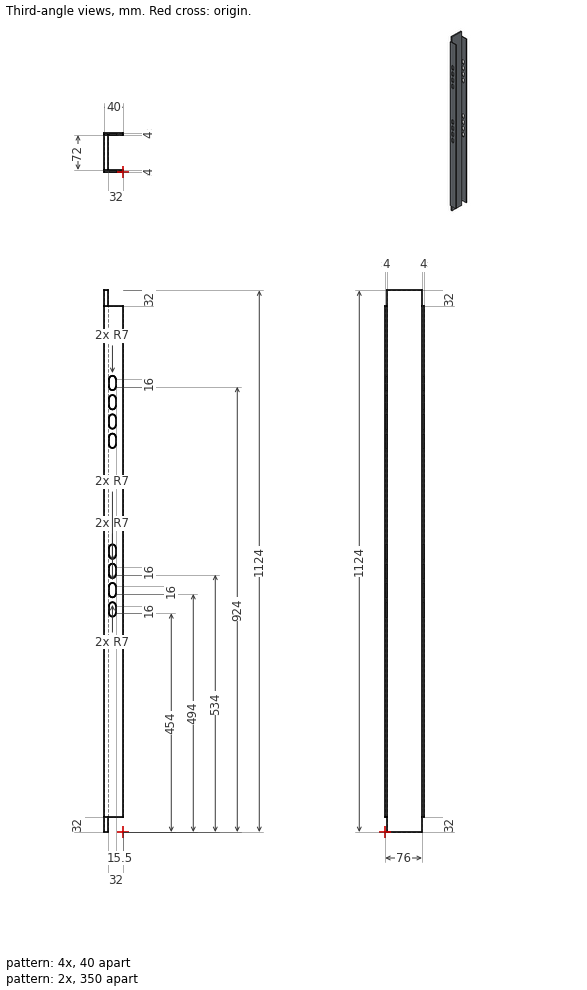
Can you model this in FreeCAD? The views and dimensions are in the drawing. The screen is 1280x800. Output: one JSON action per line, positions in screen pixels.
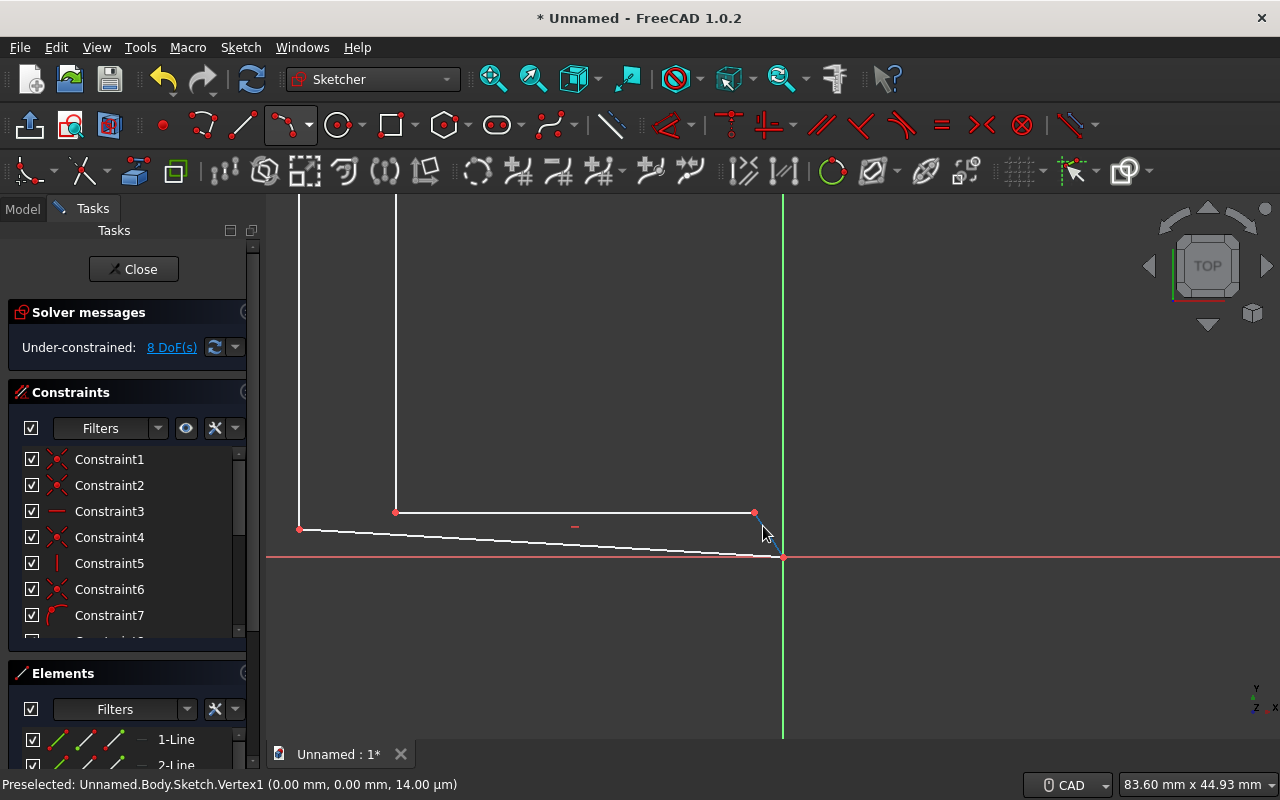
{"action": "left_click", "coordinate": [763, 526]}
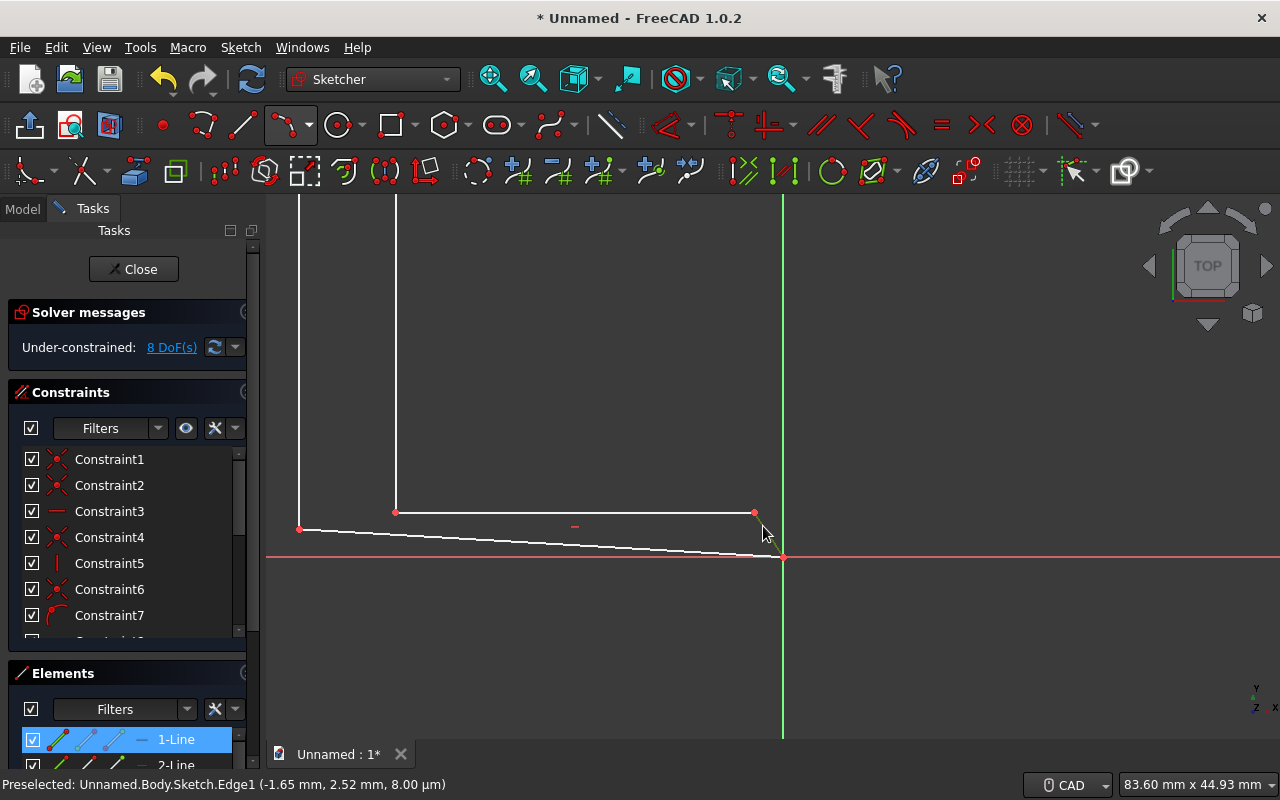
{"action": "left_click", "coordinate": [796, 126]}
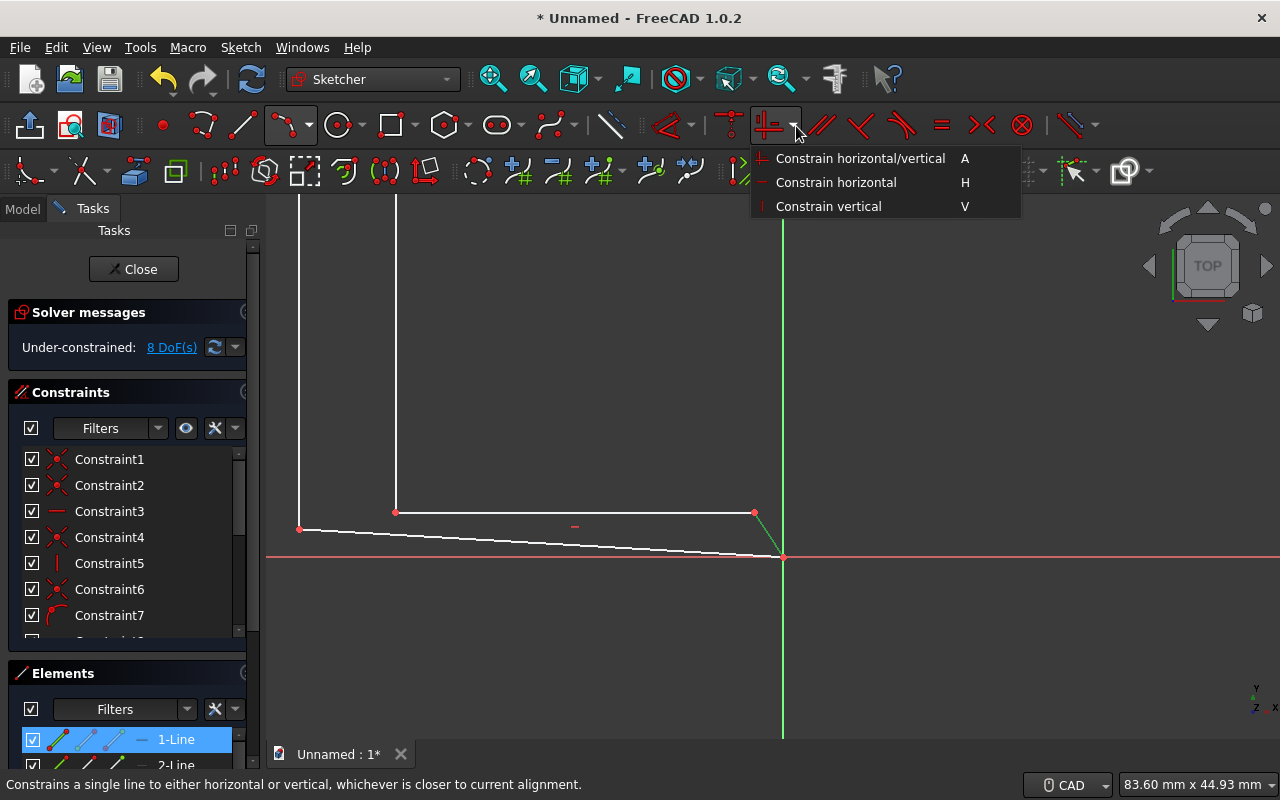
{"action": "left_click", "coordinate": [886, 206]}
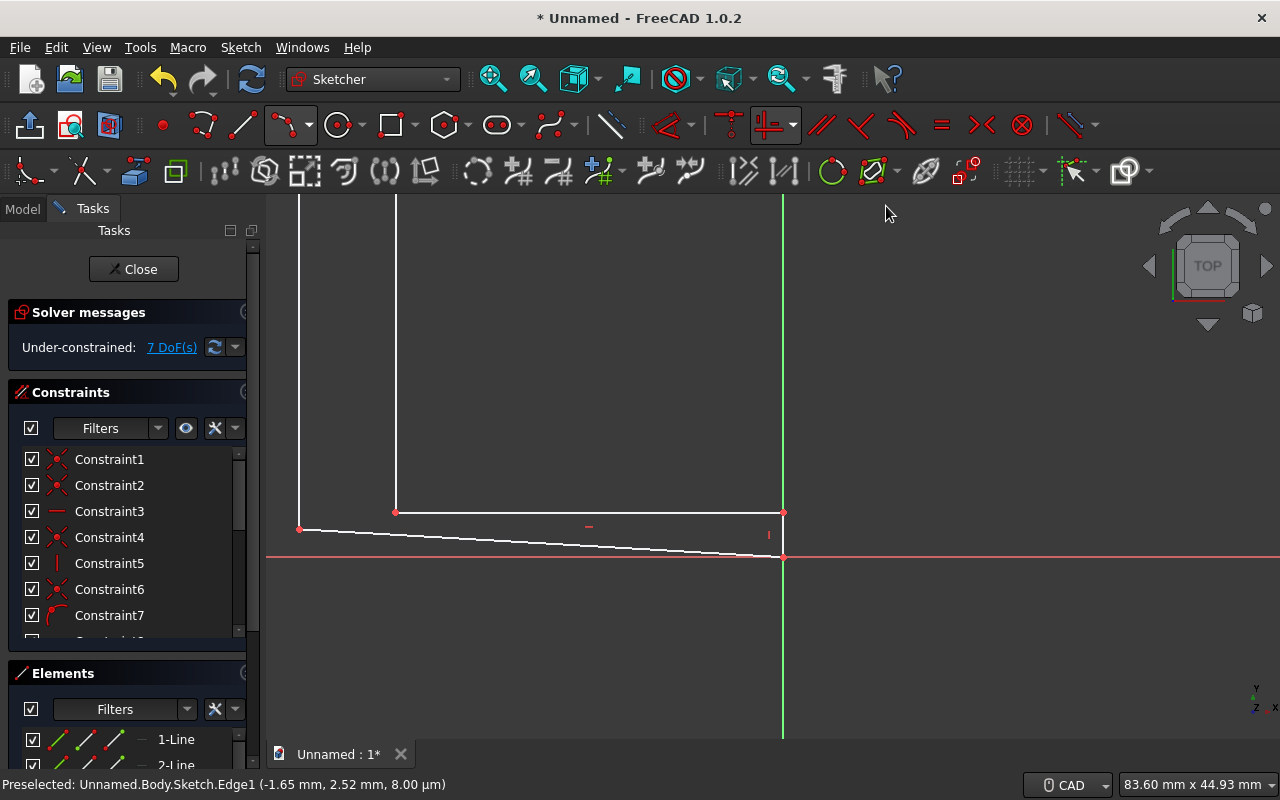
{"action": "scroll", "coordinate": [800, 696], "scroll_direction": "down", "scroll_amount": 5}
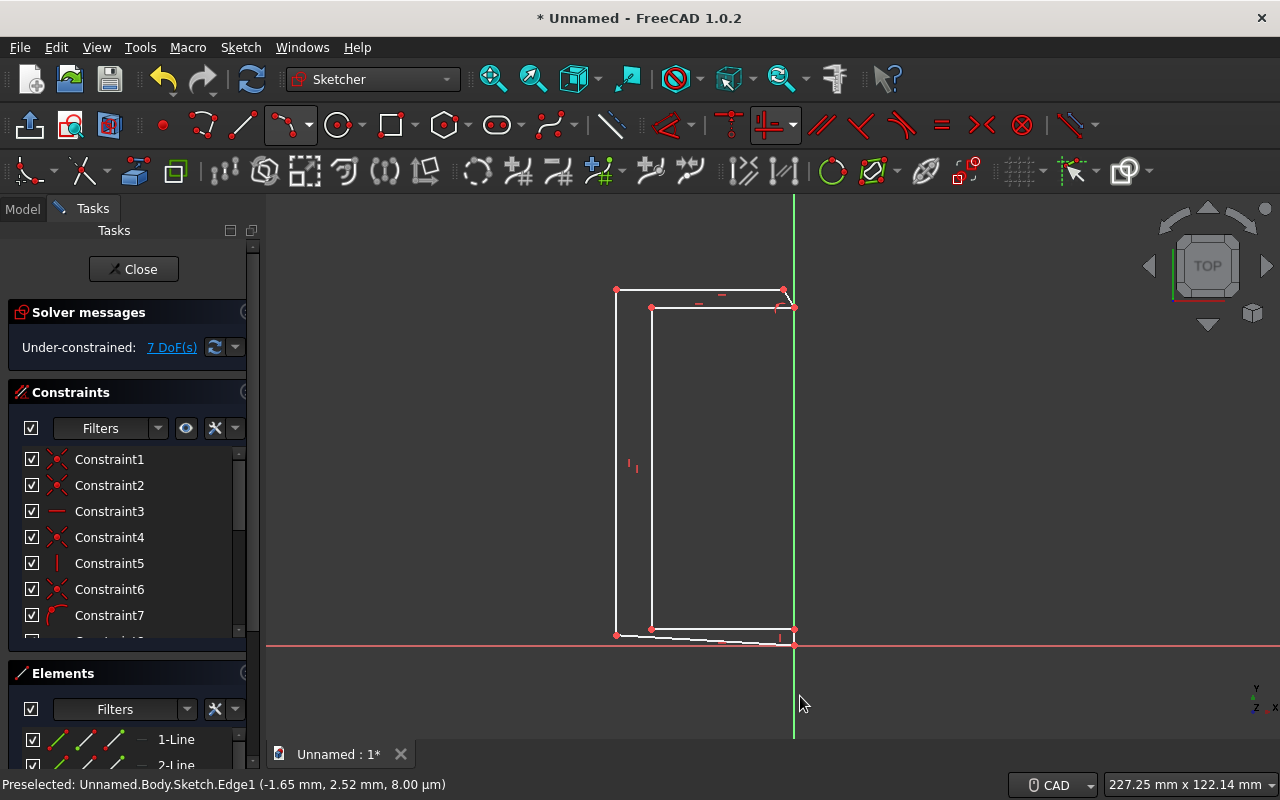
{"action": "scroll", "coordinate": [787, 295], "scroll_direction": "up", "scroll_amount": 4}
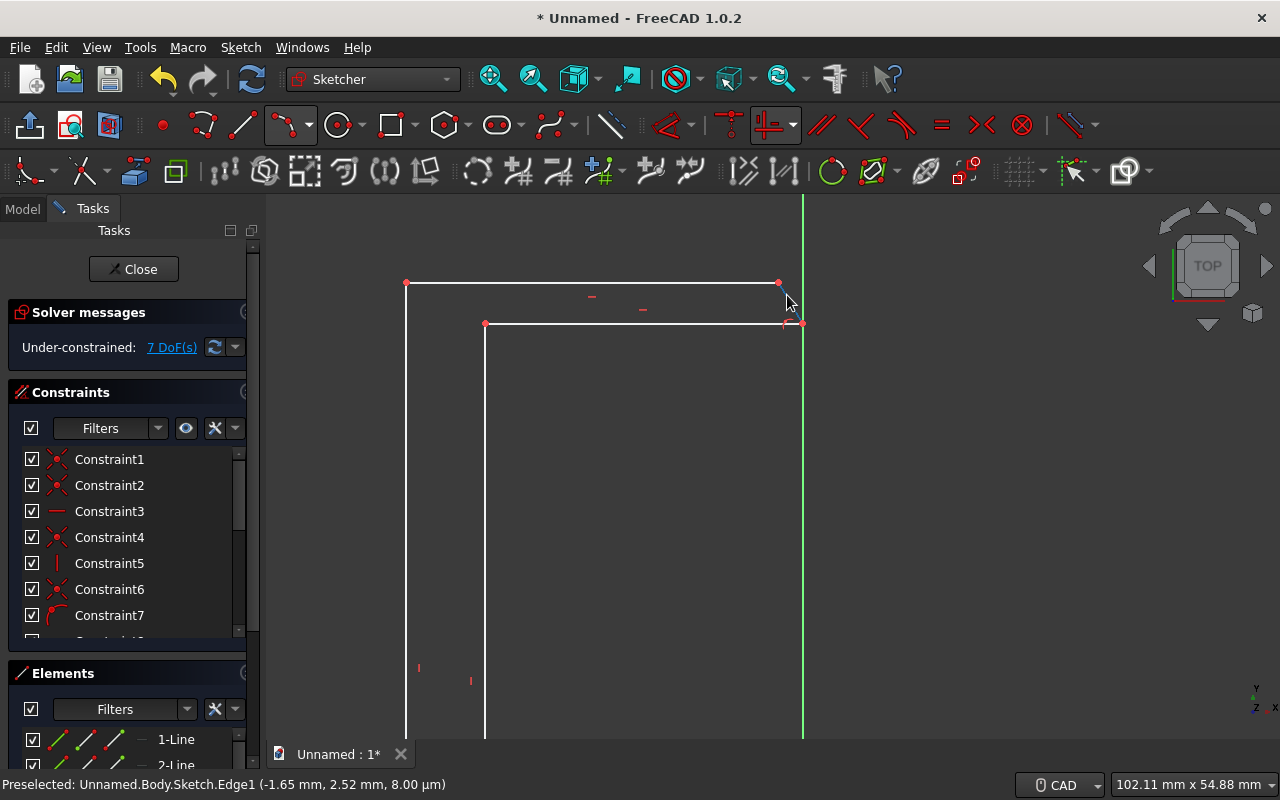
{"action": "left_click", "coordinate": [786, 295]}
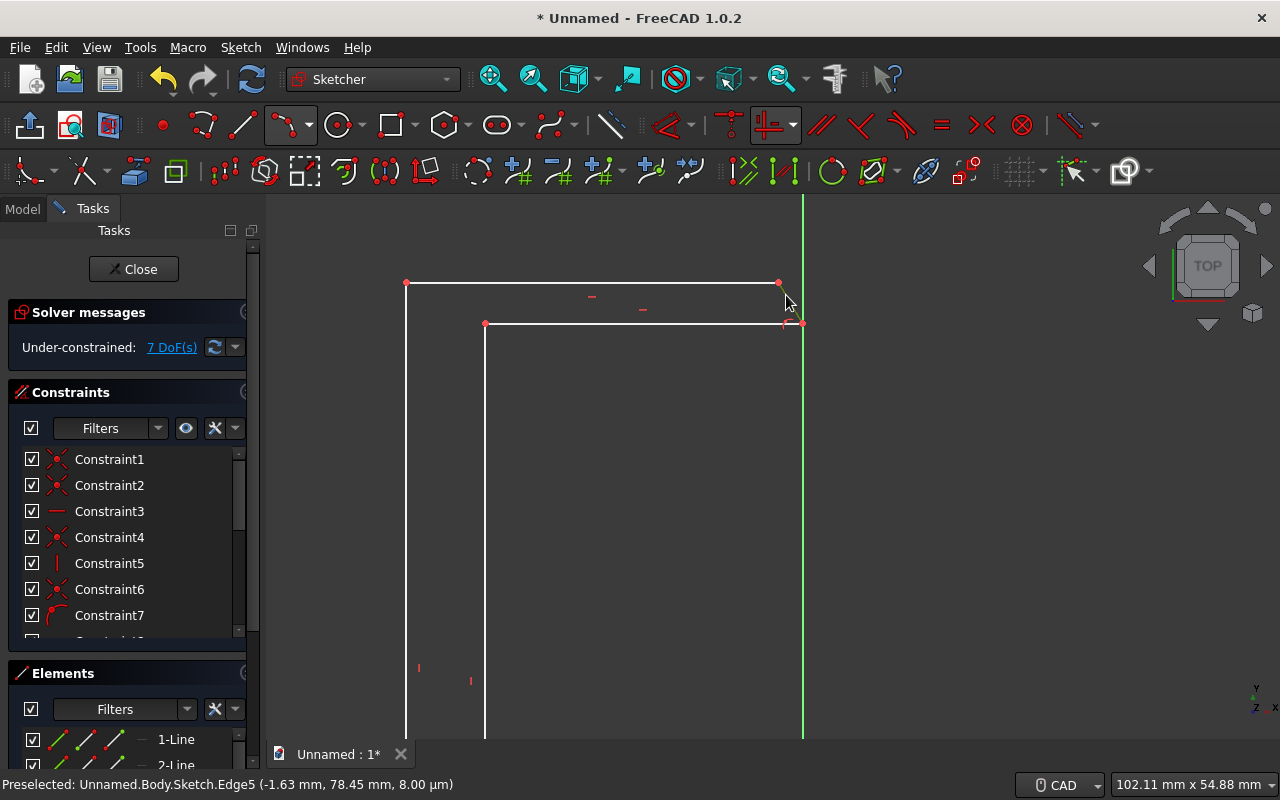
{"action": "left_click", "coordinate": [796, 126]}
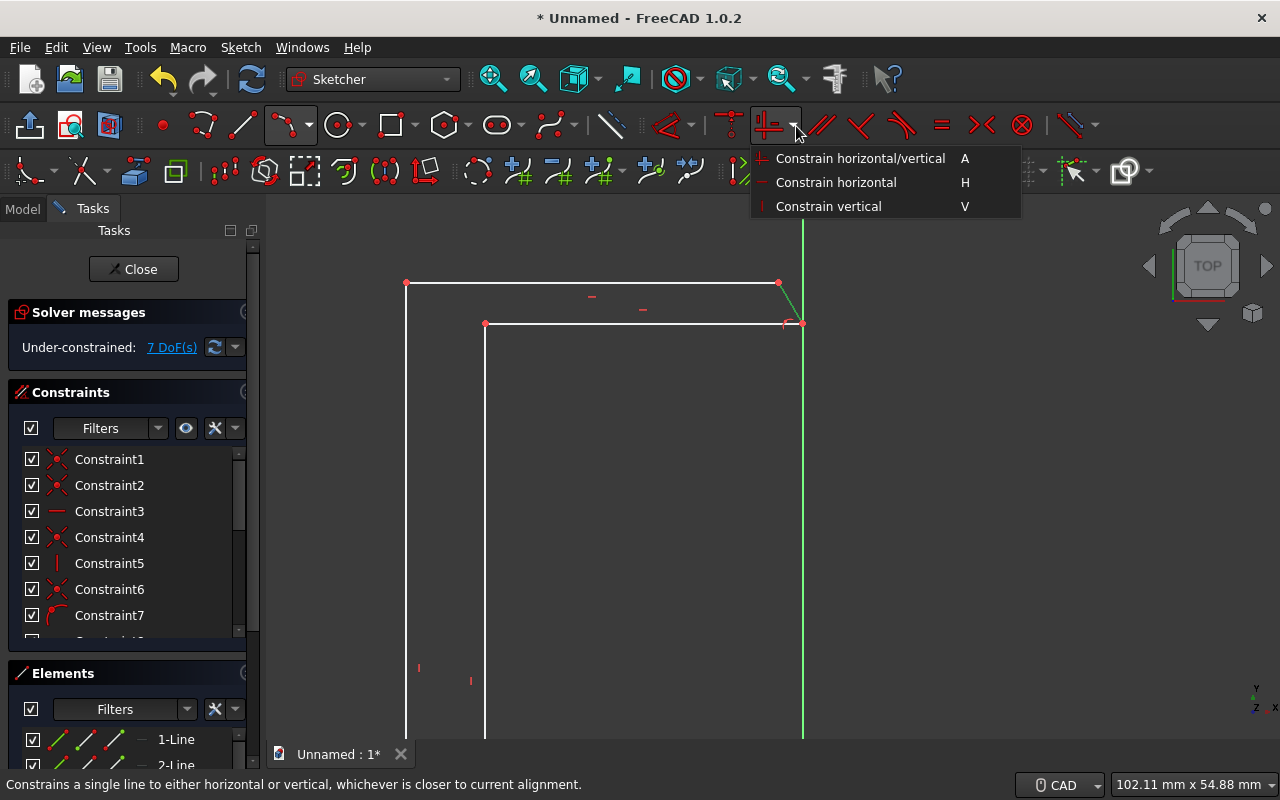
{"action": "left_click", "coordinate": [886, 206]}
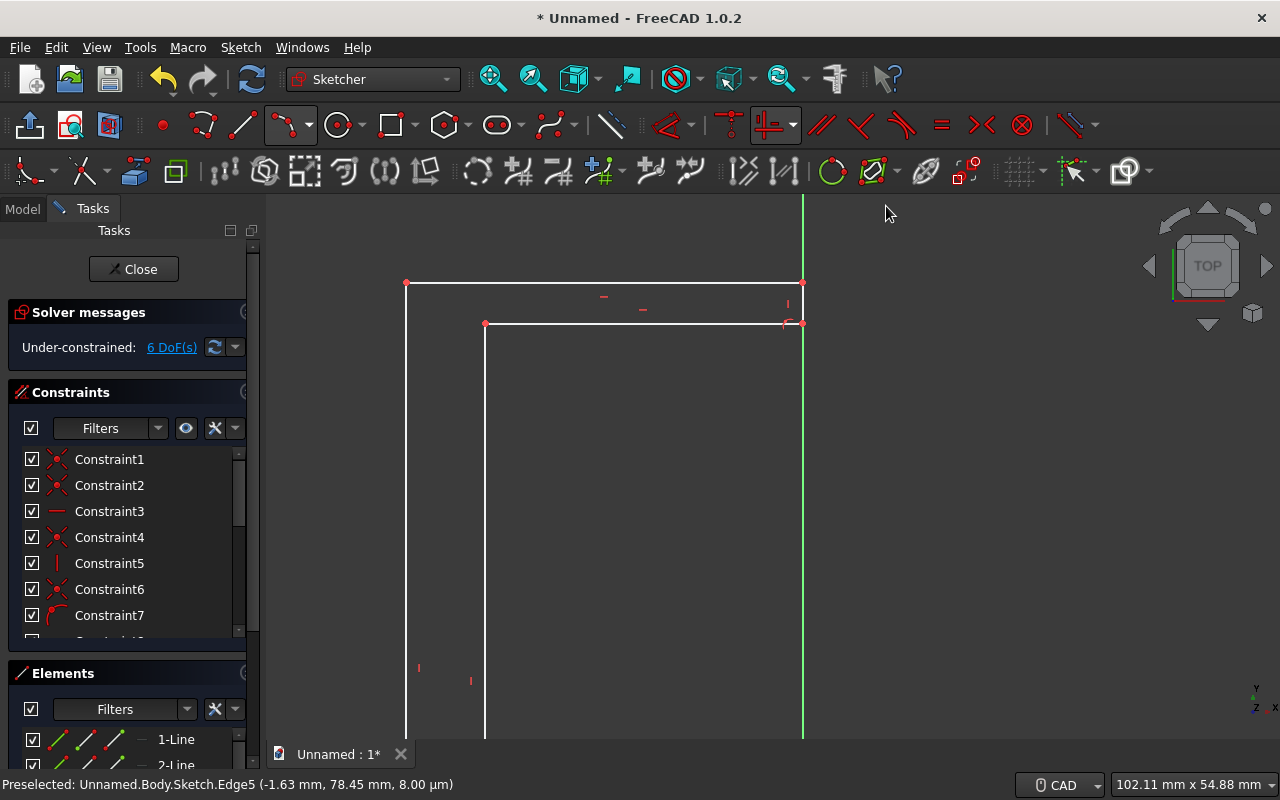
{"action": "scroll", "coordinate": [787, 294], "scroll_direction": "down", "scroll_amount": 4}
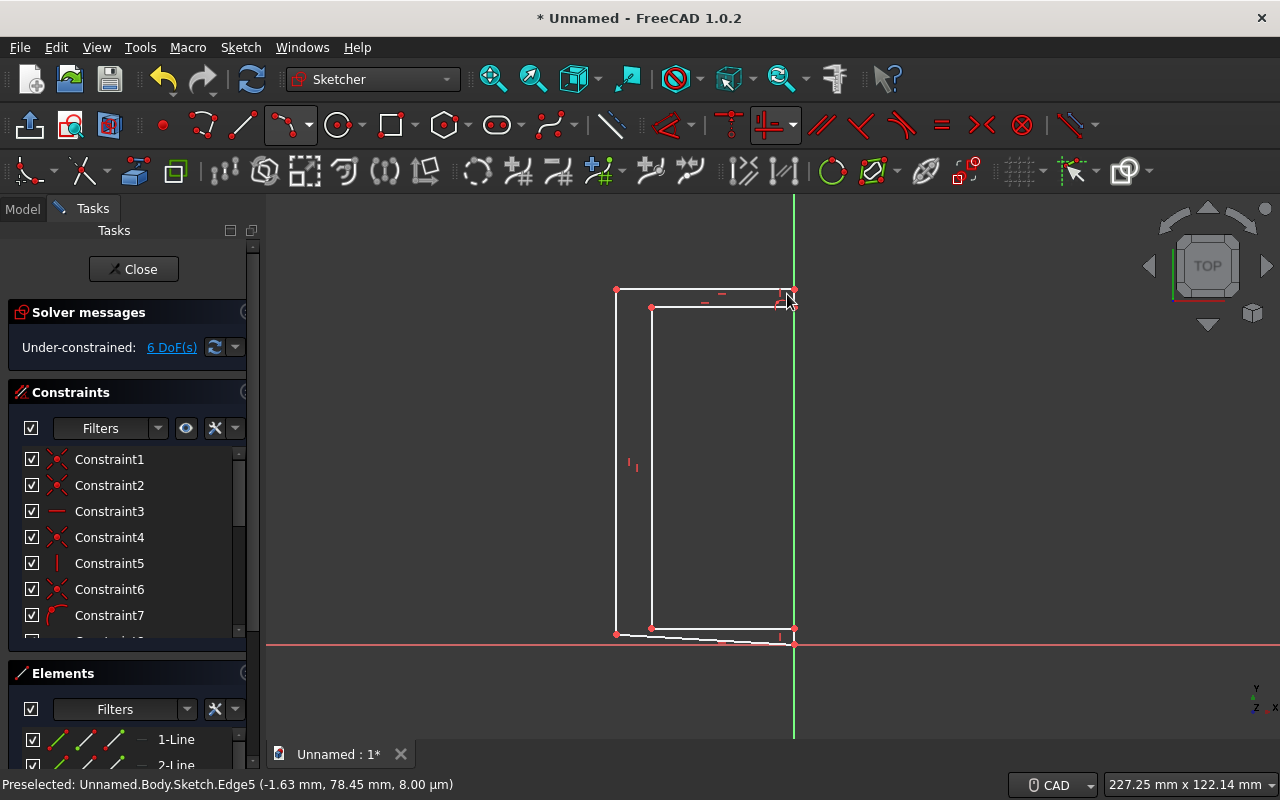
{"action": "scroll", "coordinate": [670, 638], "scroll_direction": "up", "scroll_amount": 4}